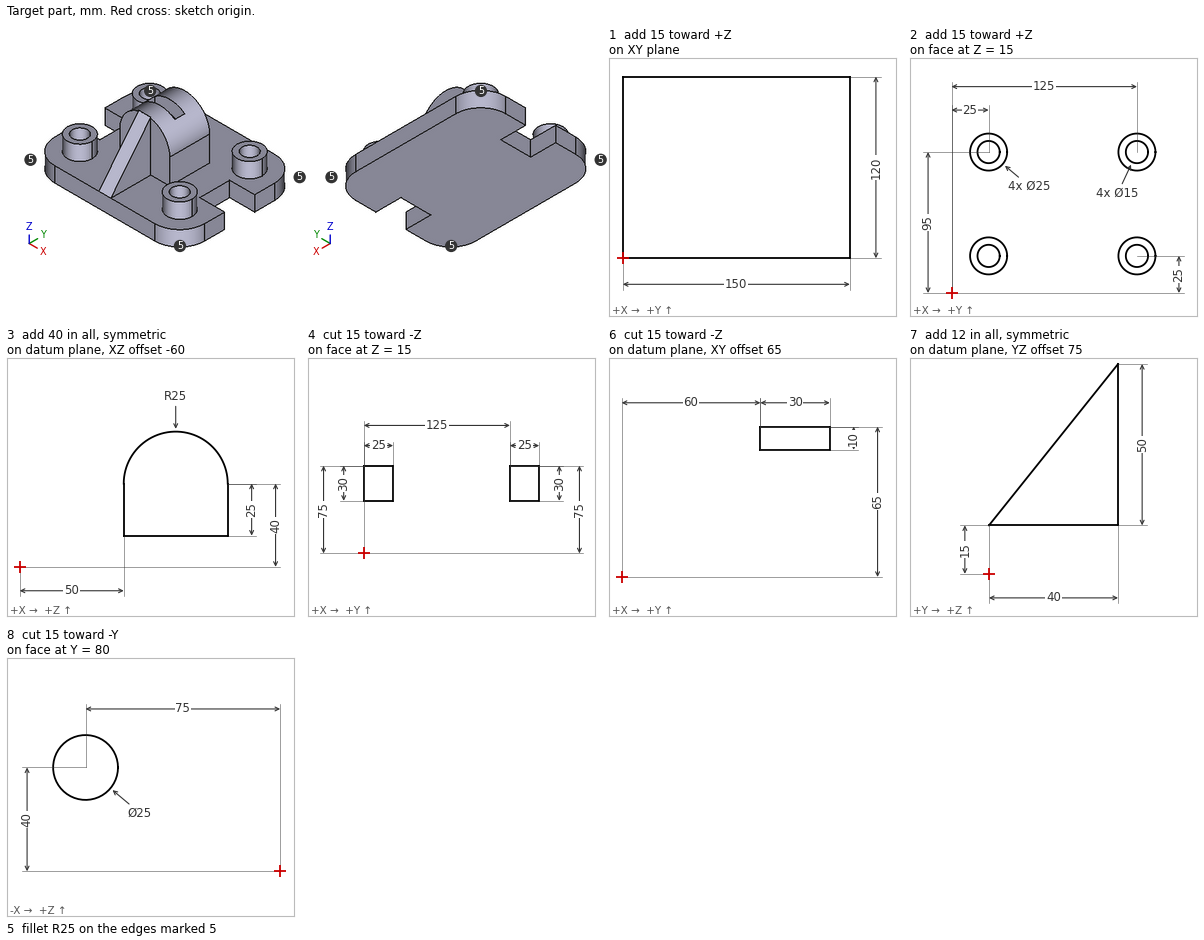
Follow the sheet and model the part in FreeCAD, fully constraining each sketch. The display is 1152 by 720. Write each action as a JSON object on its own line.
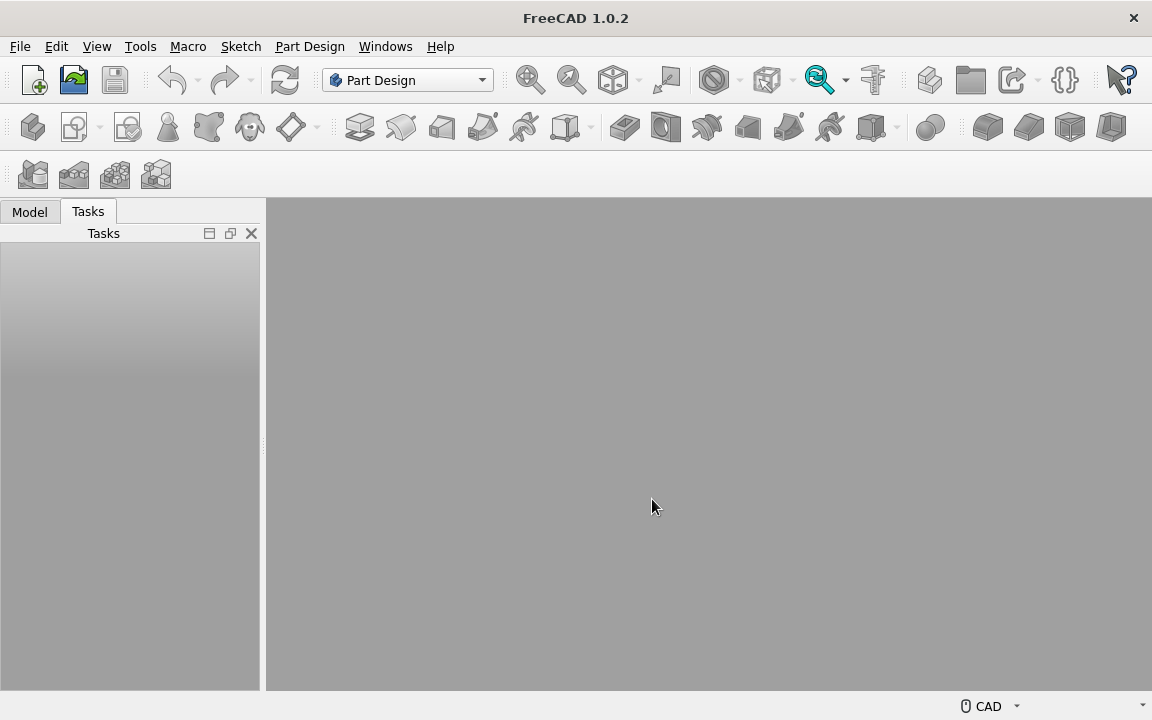
{"action": "key", "text": "ctrl+n"}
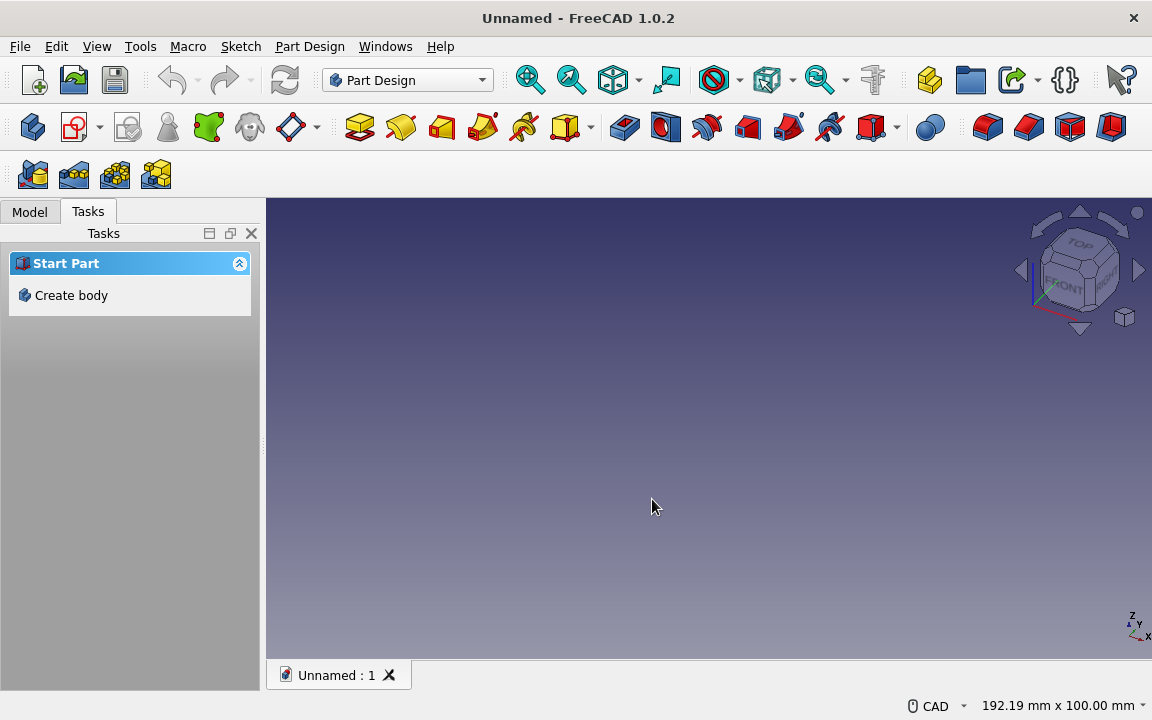
{"action": "left_click", "coordinate": [74, 128]}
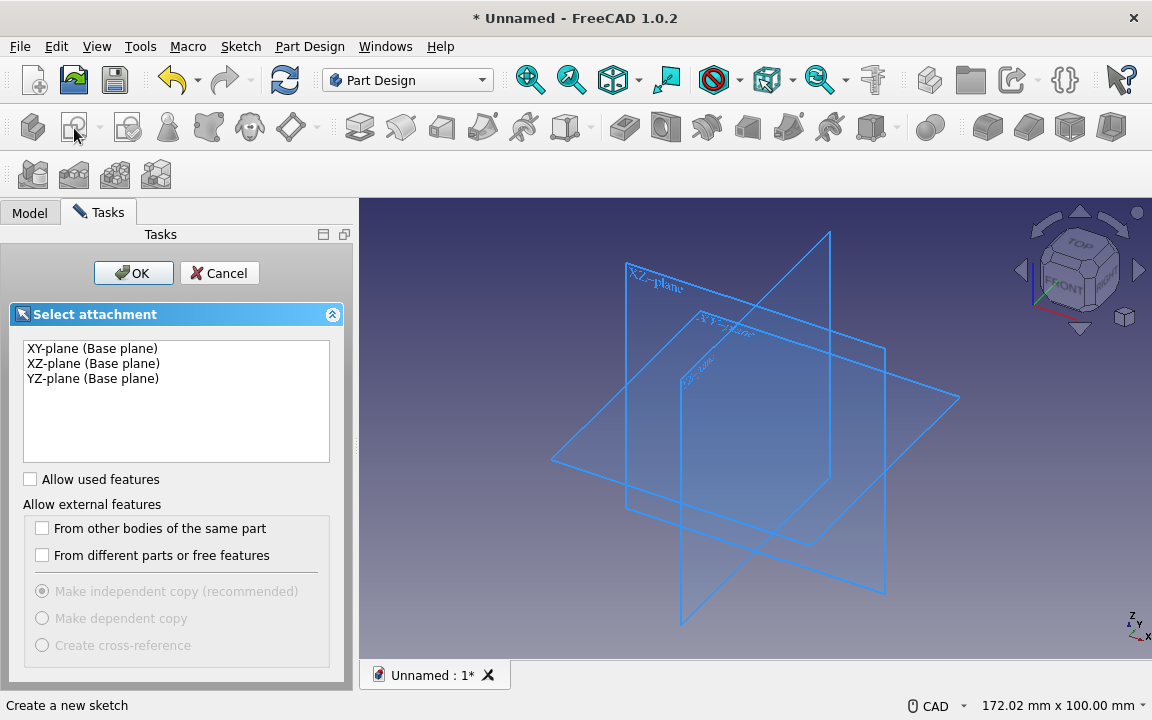
{"action": "left_click", "coordinate": [84, 348]}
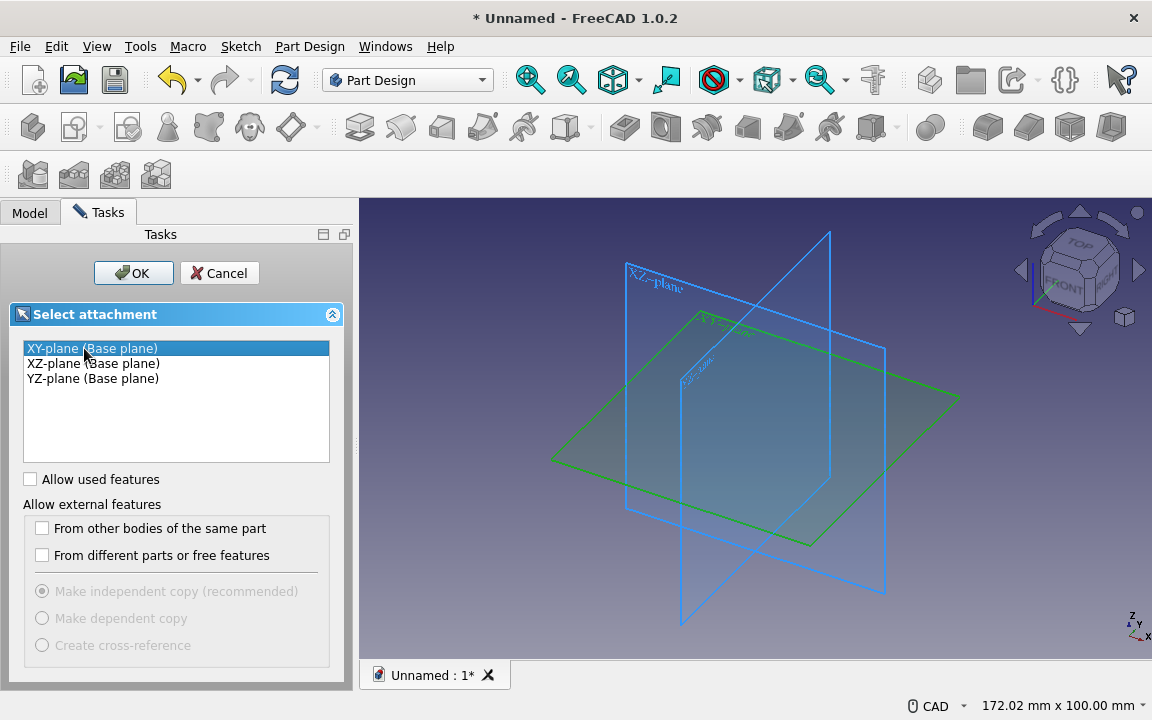
{"action": "left_click", "coordinate": [134, 273]}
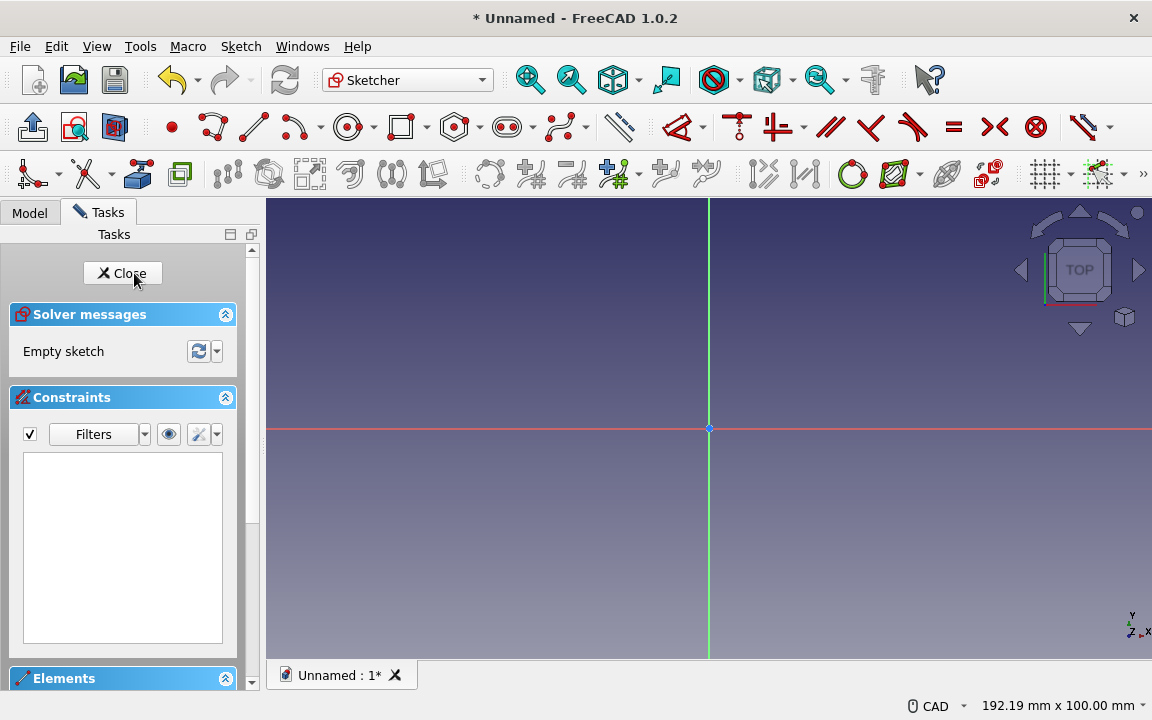
{"action": "scroll", "coordinate": [302, 631], "scroll_direction": "down", "scroll_amount": 4}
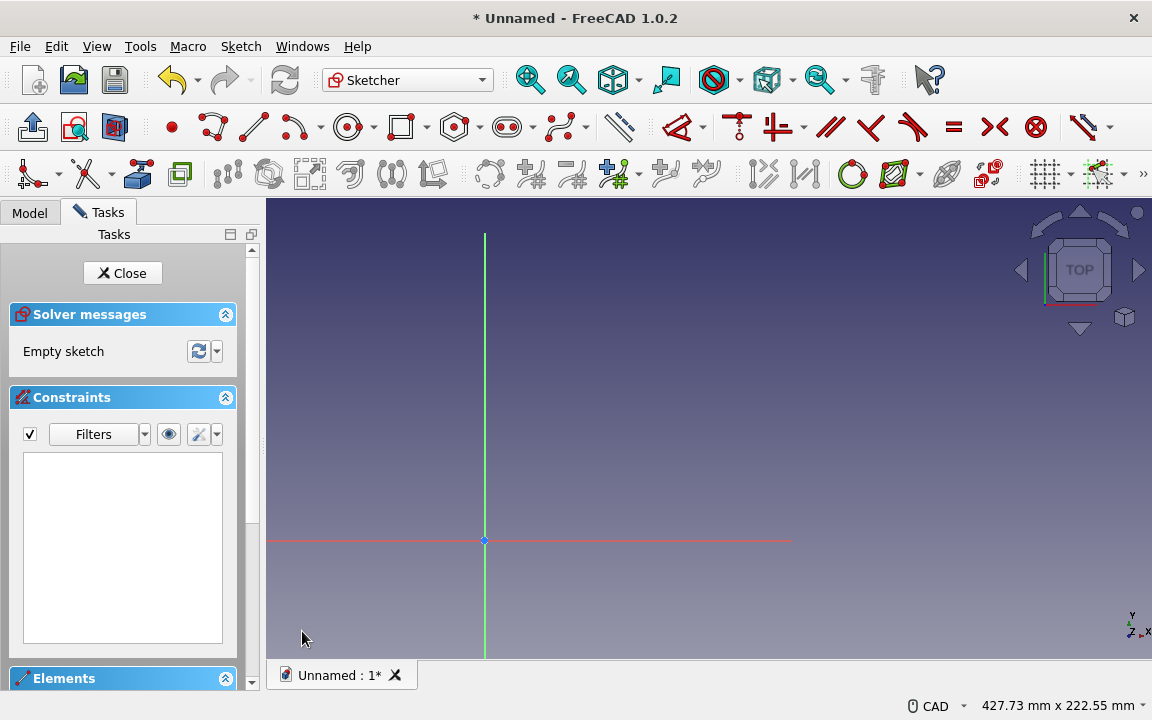
{"action": "left_click", "coordinate": [400, 128]}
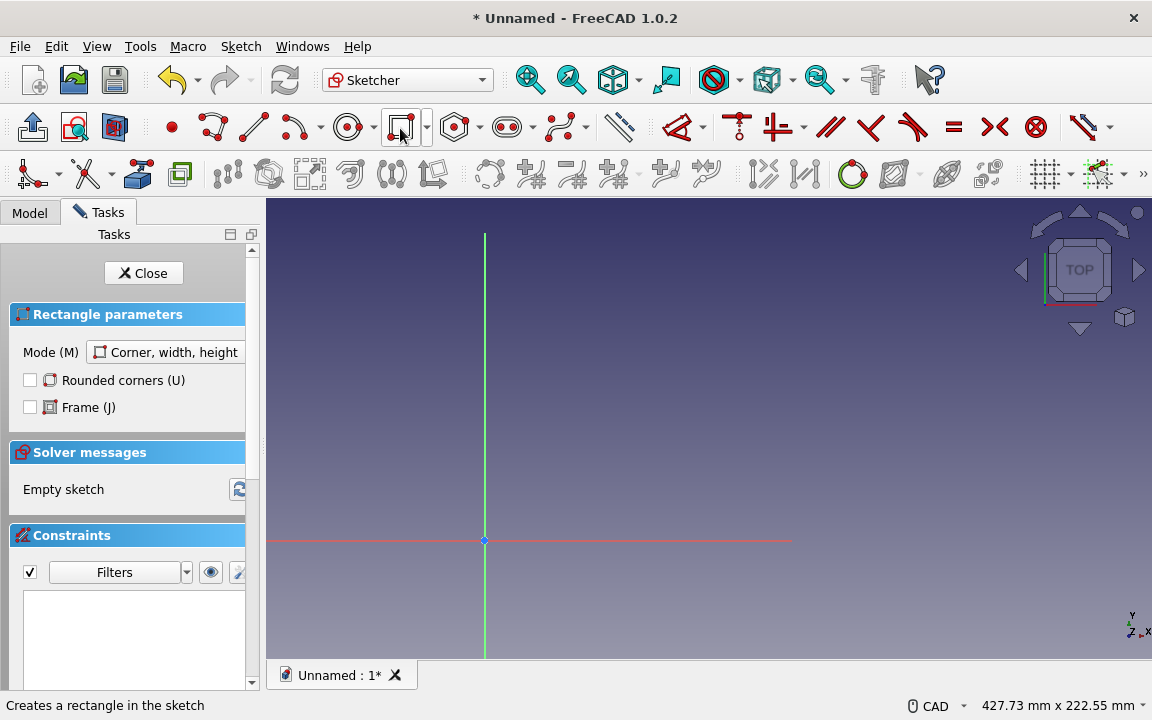
{"action": "left_click", "coordinate": [485, 541]}
{"action": "left_click", "coordinate": [796, 292]}
{"action": "key", "text": "Escape"}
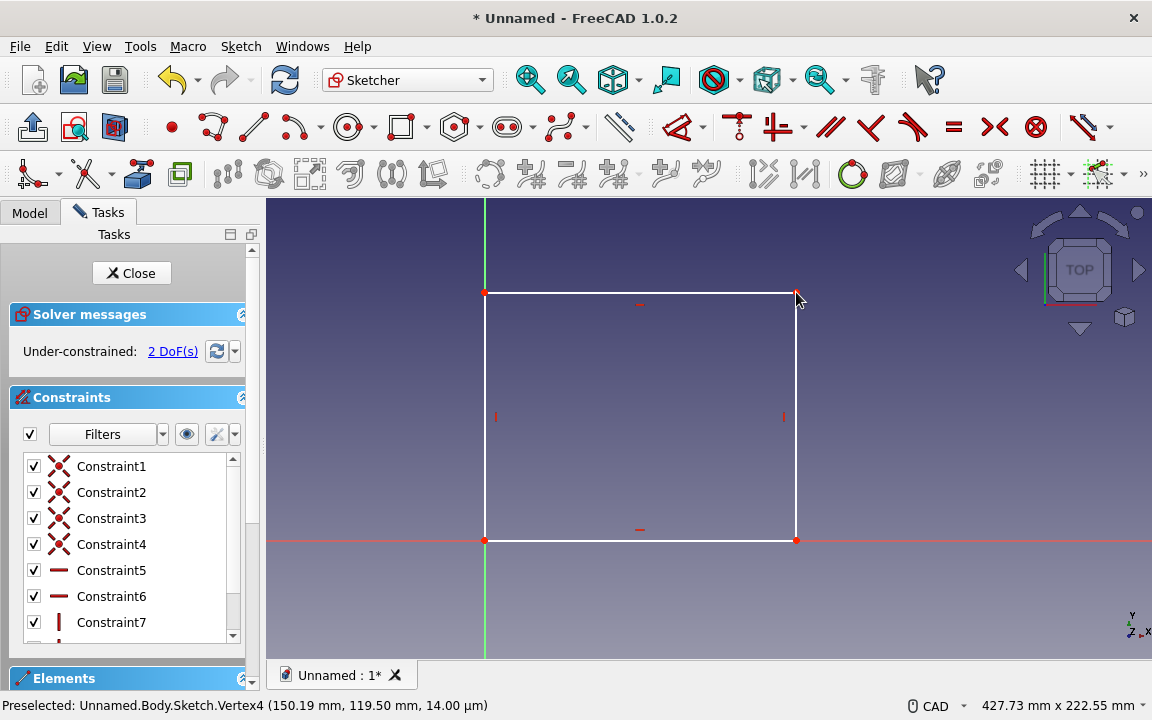
{"action": "left_click", "coordinate": [676, 128]}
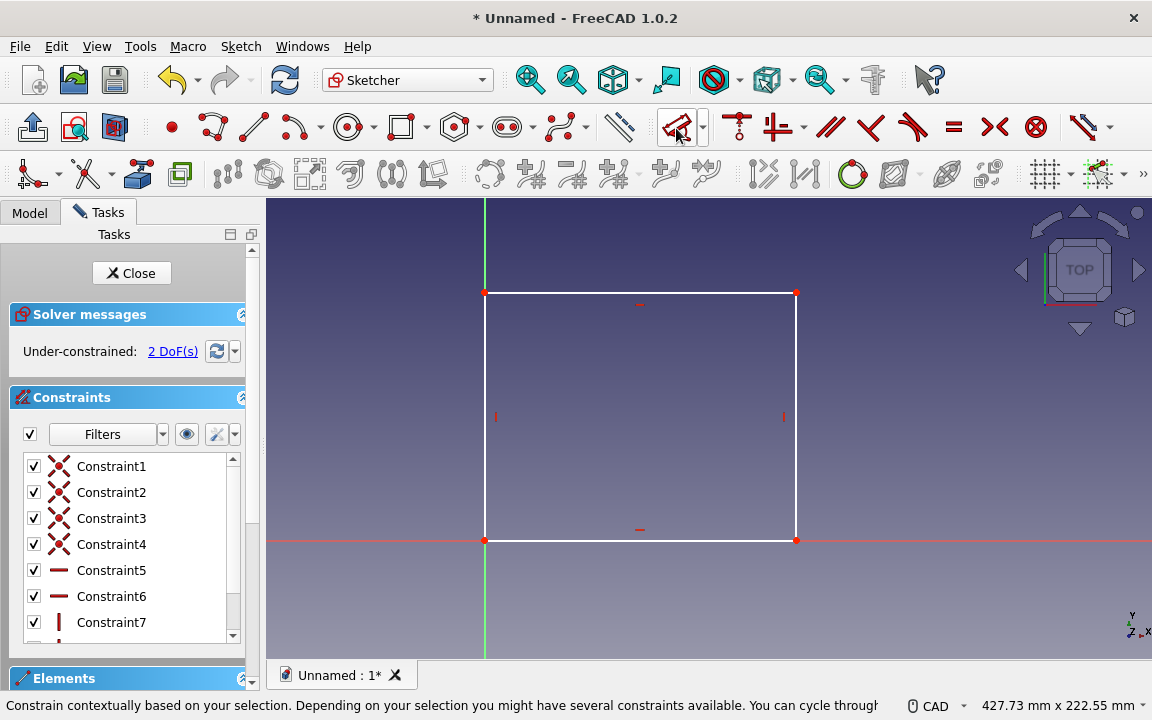
{"action": "left_click", "coordinate": [578, 541]}
{"action": "left_click", "coordinate": [640, 575]}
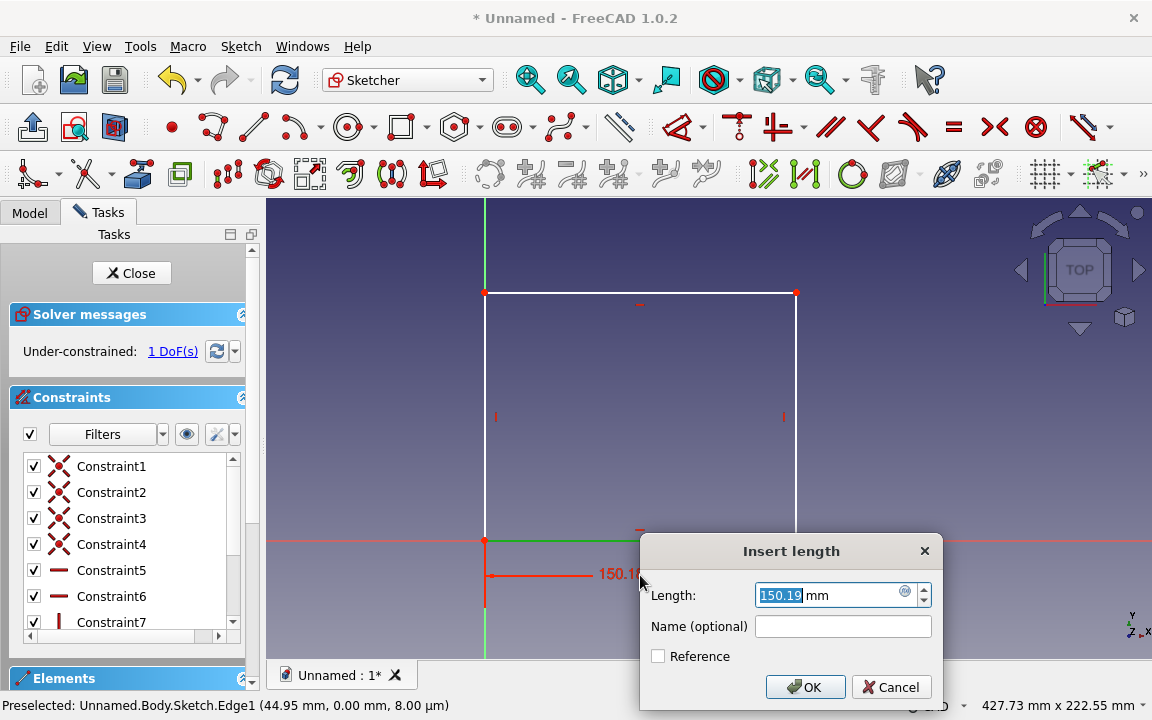
{"action": "type", "text": "150"}
{"action": "key", "text": "Return"}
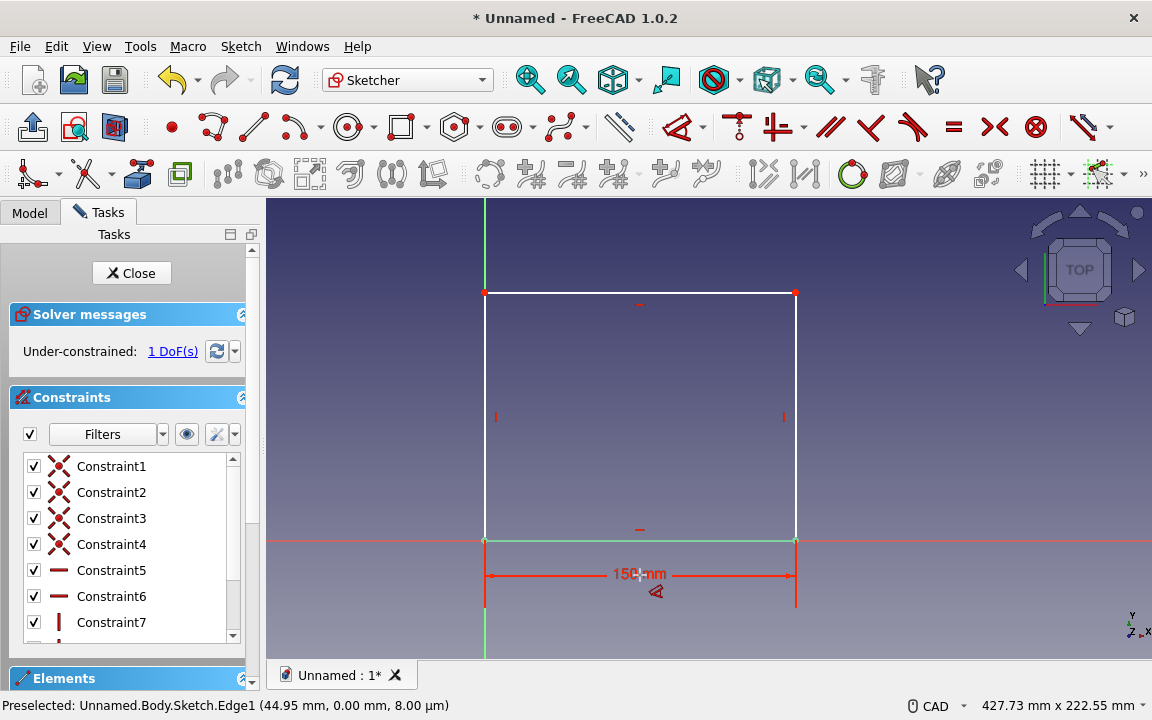
{"action": "left_click", "coordinate": [796, 466]}
{"action": "left_click", "coordinate": [830, 417]}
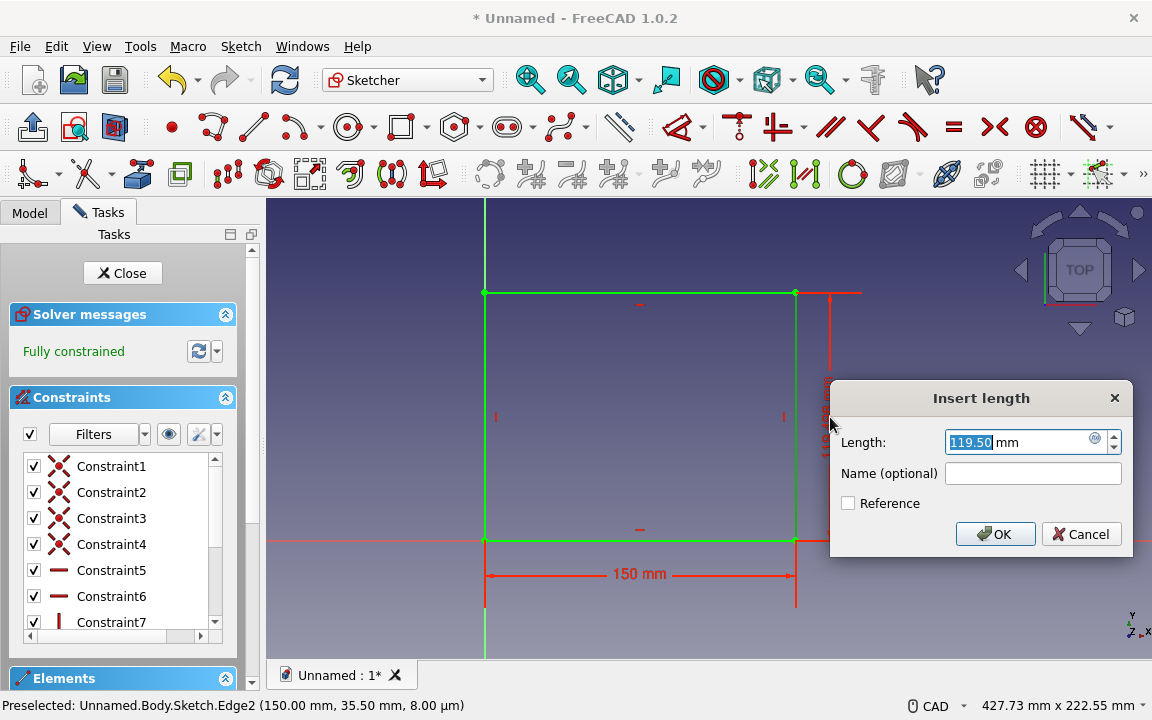
{"action": "type", "text": "120"}
{"action": "key", "text": "Return"}
{"action": "key", "text": "Escape"}